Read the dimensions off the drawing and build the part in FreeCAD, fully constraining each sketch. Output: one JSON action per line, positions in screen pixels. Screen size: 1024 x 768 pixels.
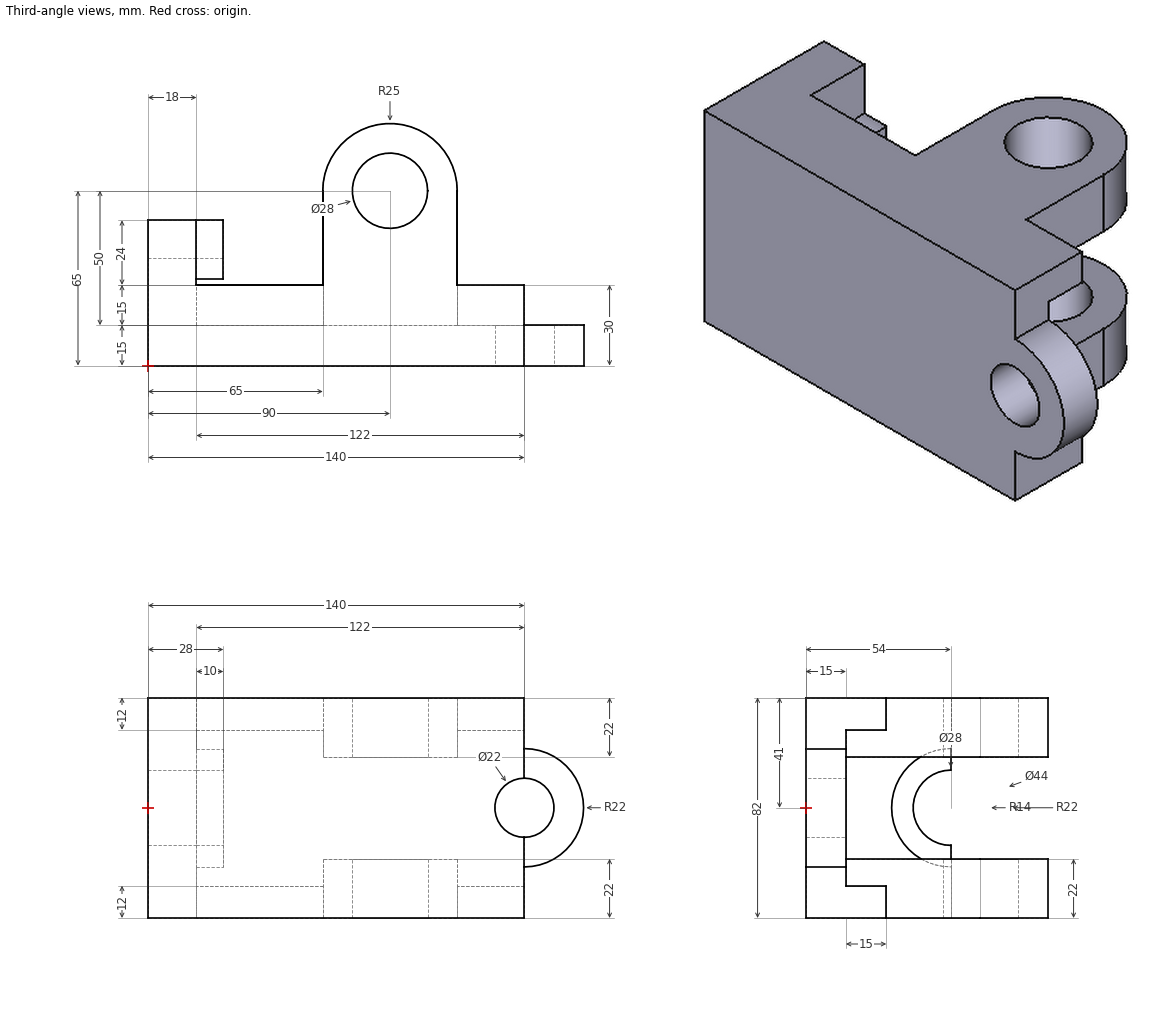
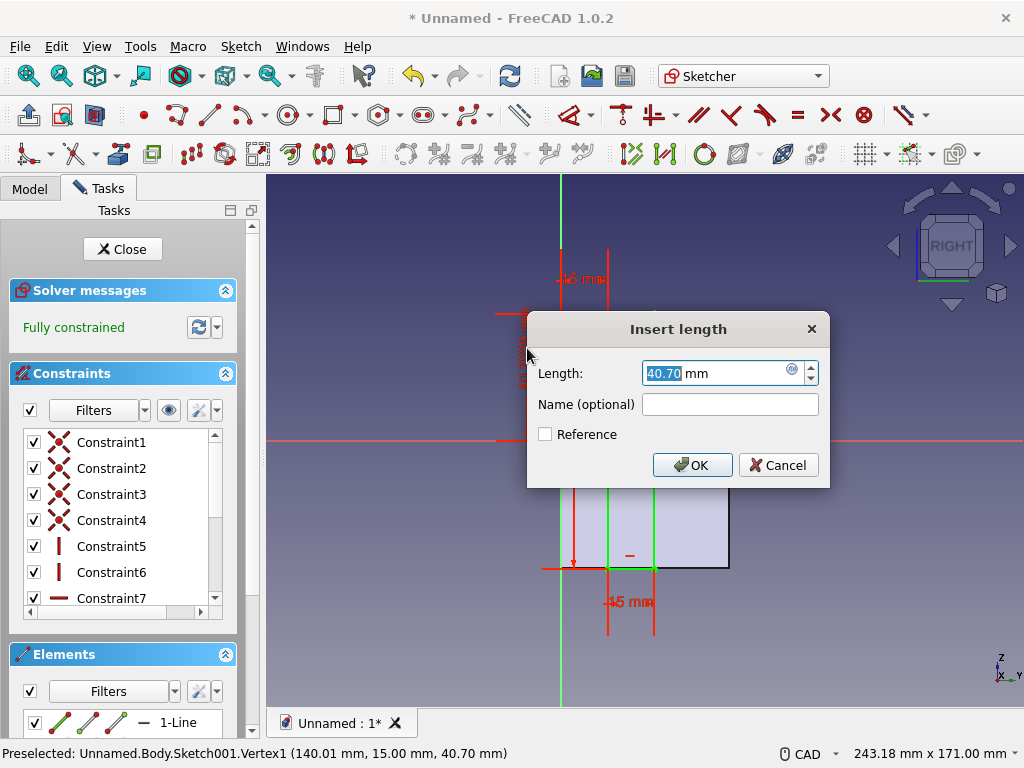
{"action": "type", "text": "41"}
{"action": "key", "text": "Return"}
{"action": "key", "text": "Escape"}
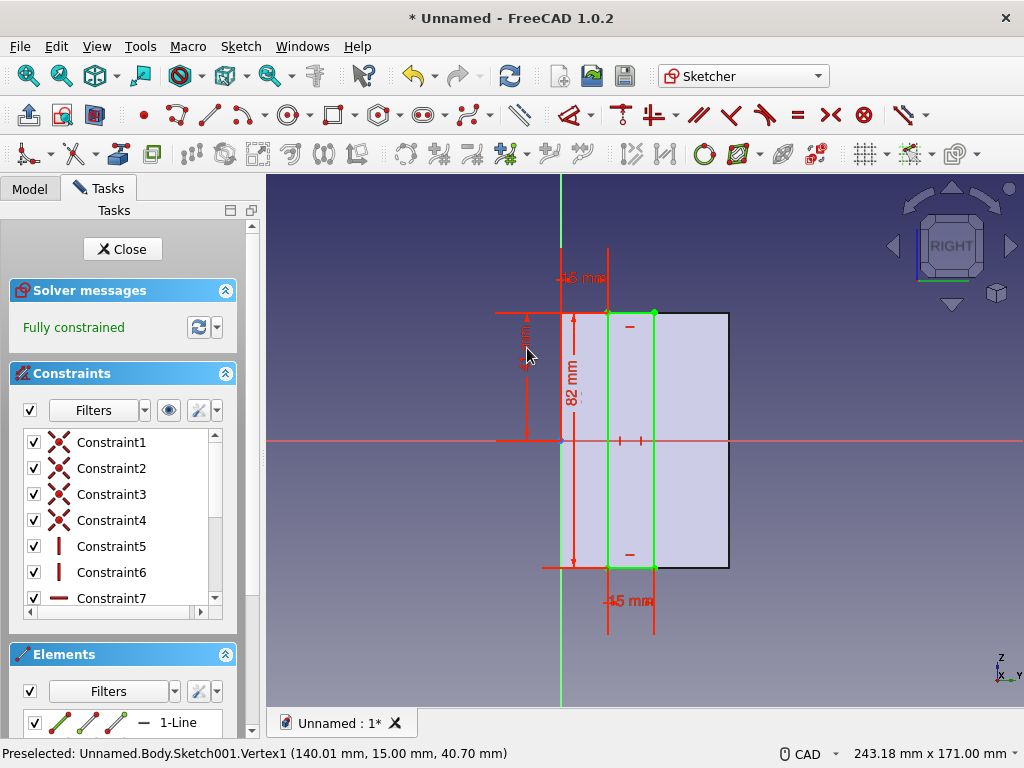
{"action": "left_click", "coordinate": [123, 249]}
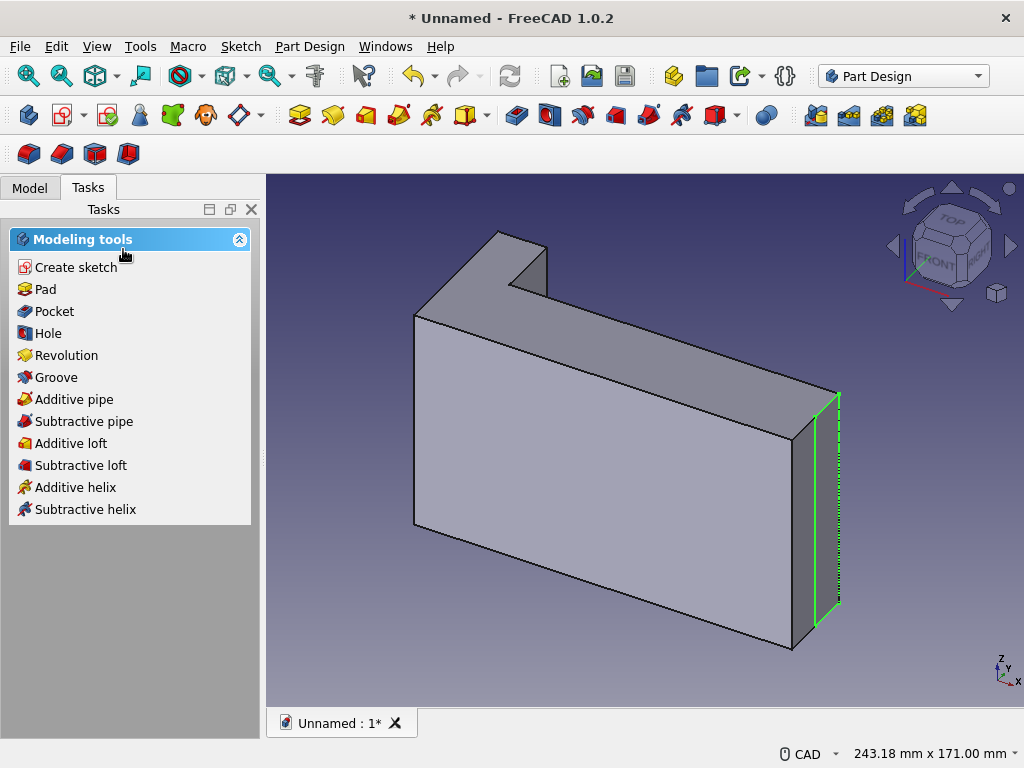
{"action": "left_click", "coordinate": [517, 116]}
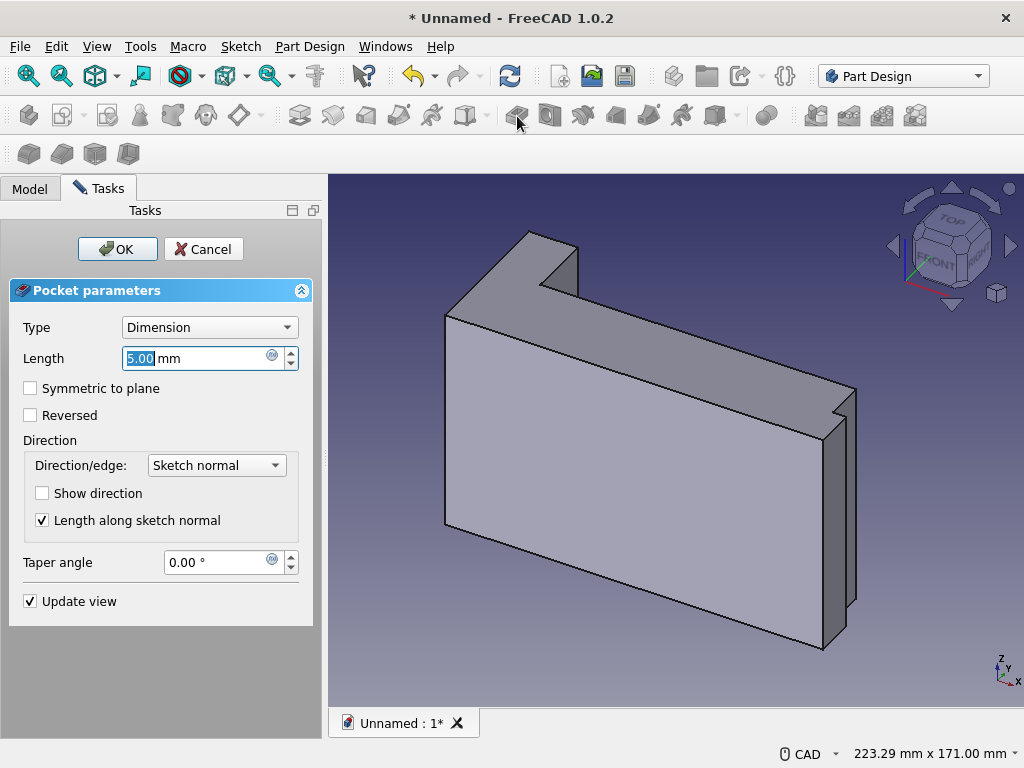
{"action": "type", "text": "122"}
{"action": "key", "text": "Tab"}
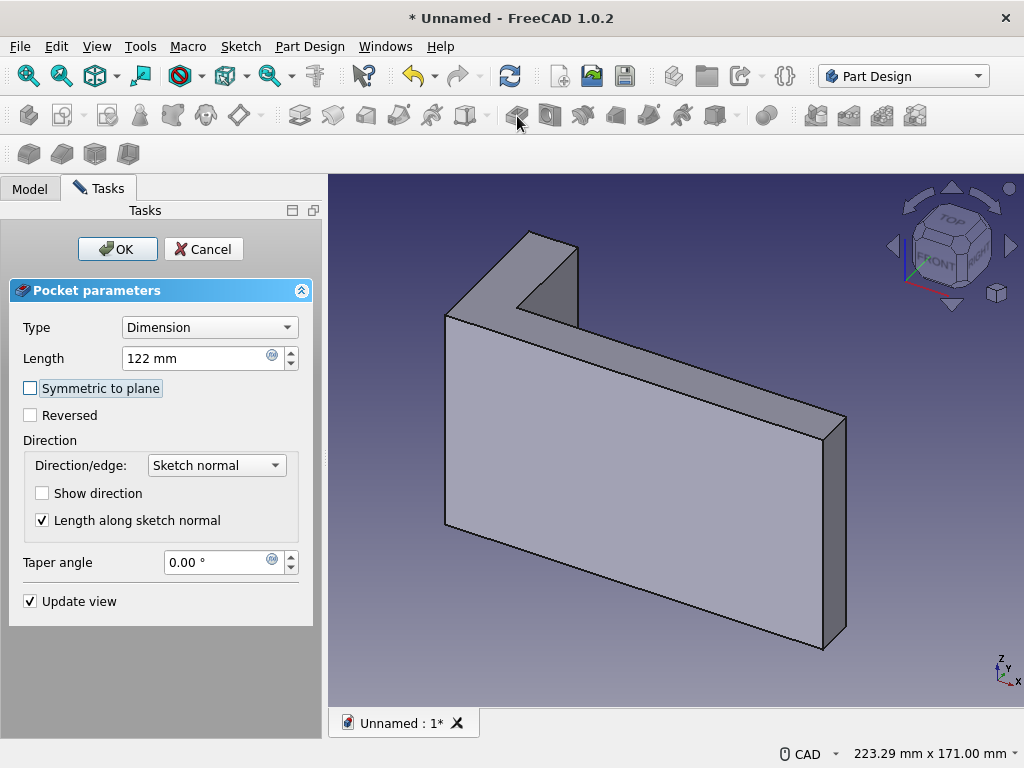
{"action": "left_click", "coordinate": [118, 249]}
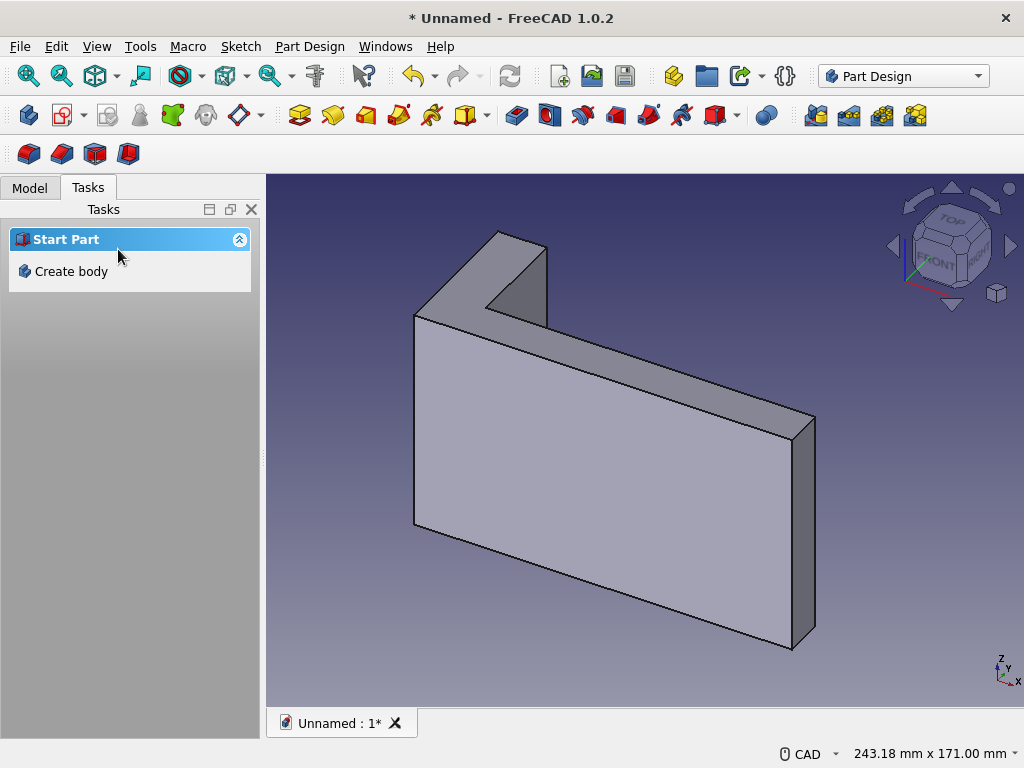
{"action": "left_click", "coordinate": [459, 305]}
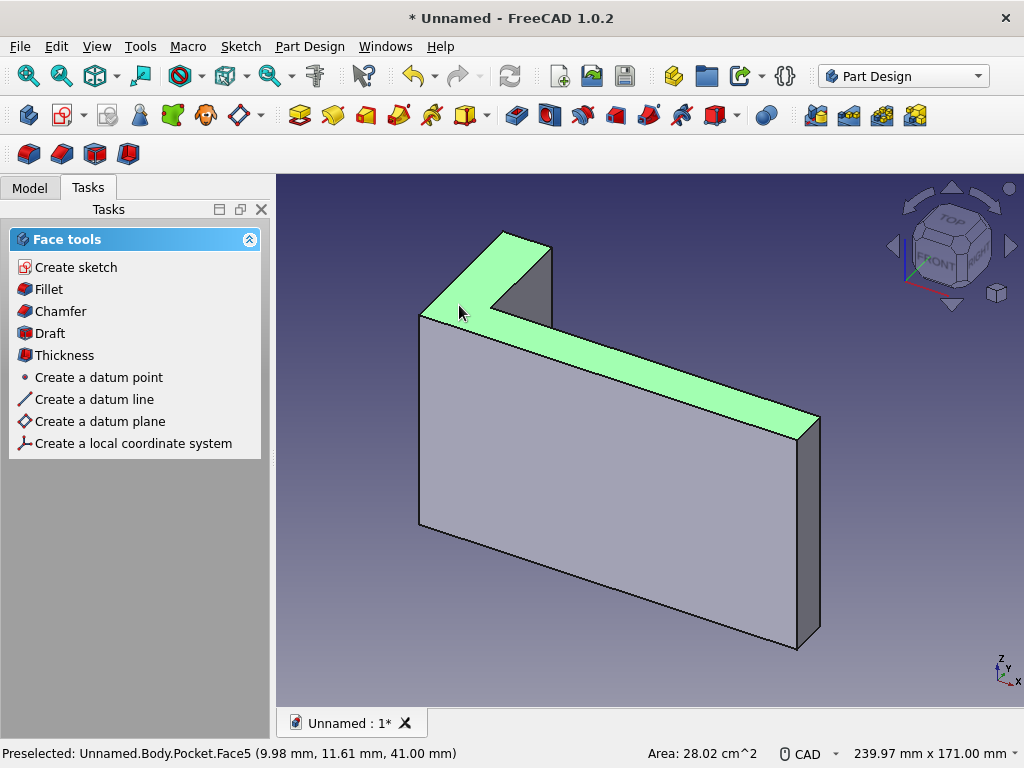
{"action": "left_click", "coordinate": [62, 116]}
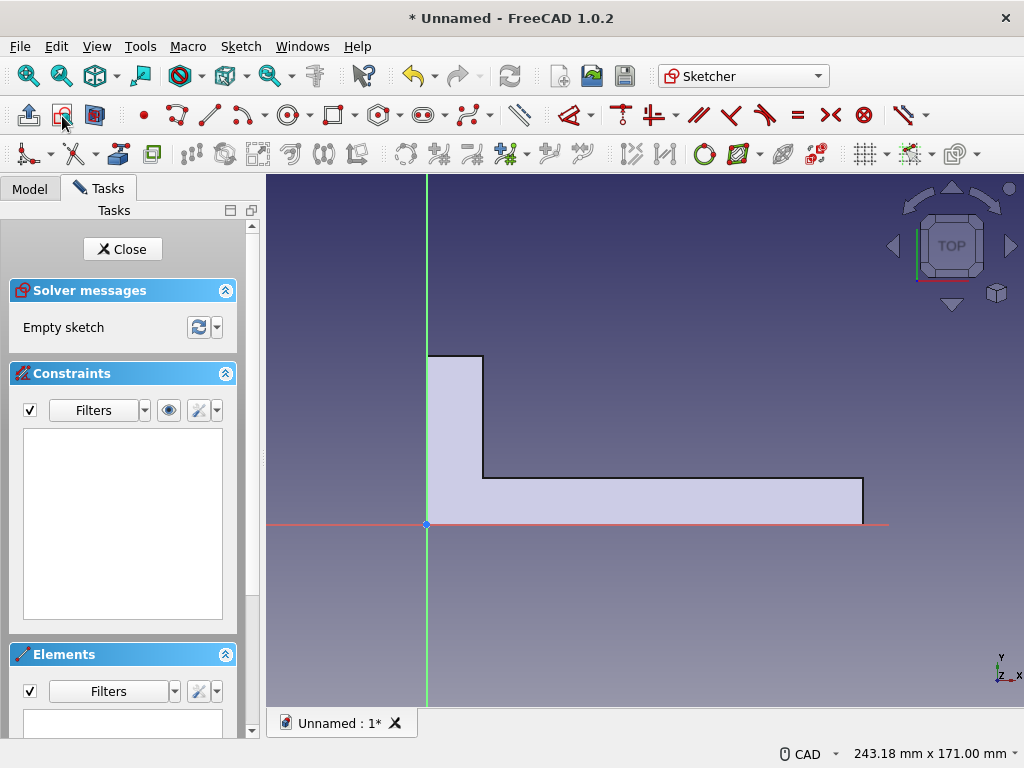
{"action": "scroll", "coordinate": [294, 272], "scroll_direction": "down", "scroll_amount": 1}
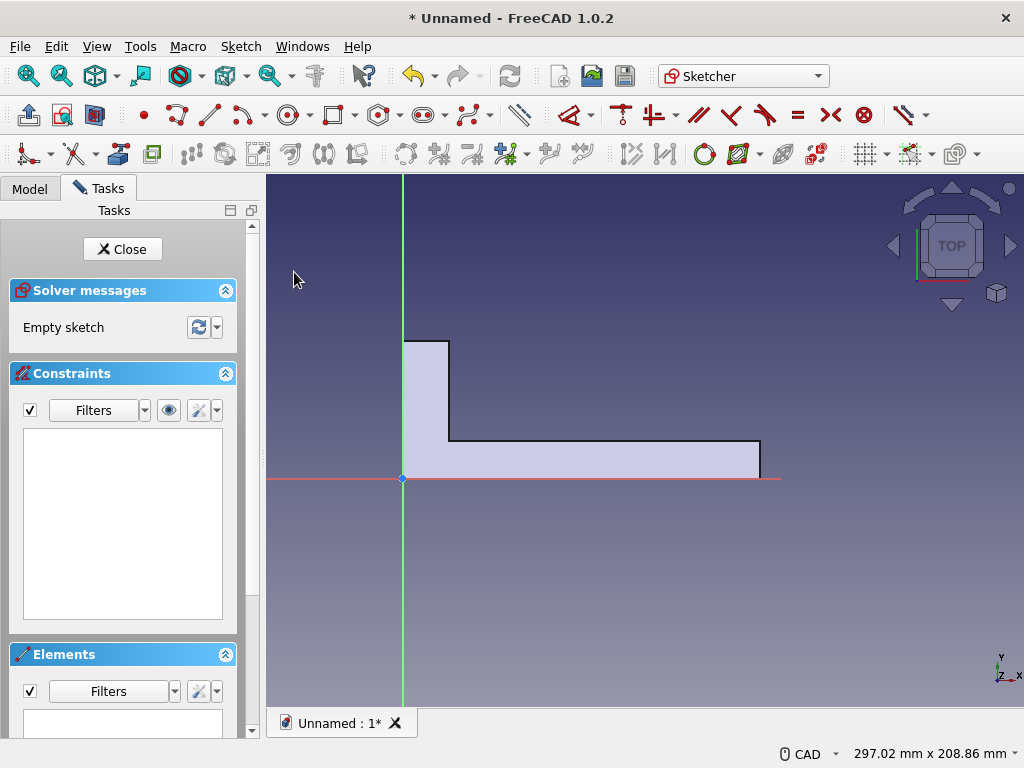
{"action": "key", "text": "g r"}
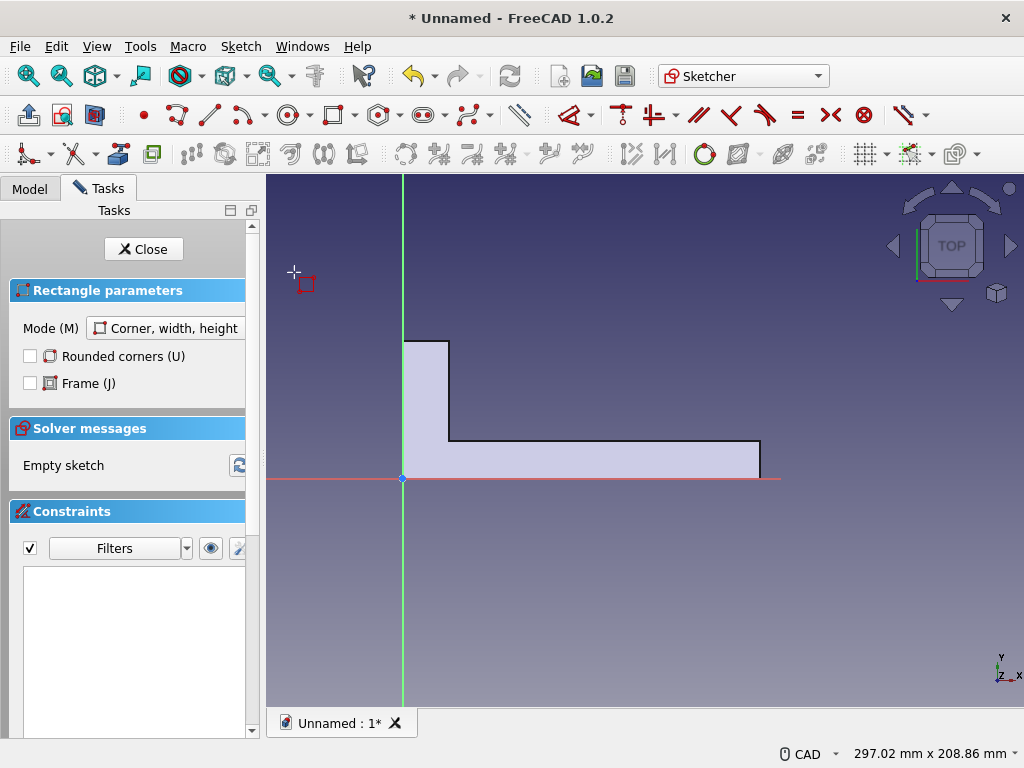
{"action": "left_click", "coordinate": [449, 402]}
{"action": "left_click", "coordinate": [760, 441]}
{"action": "key", "text": "Escape"}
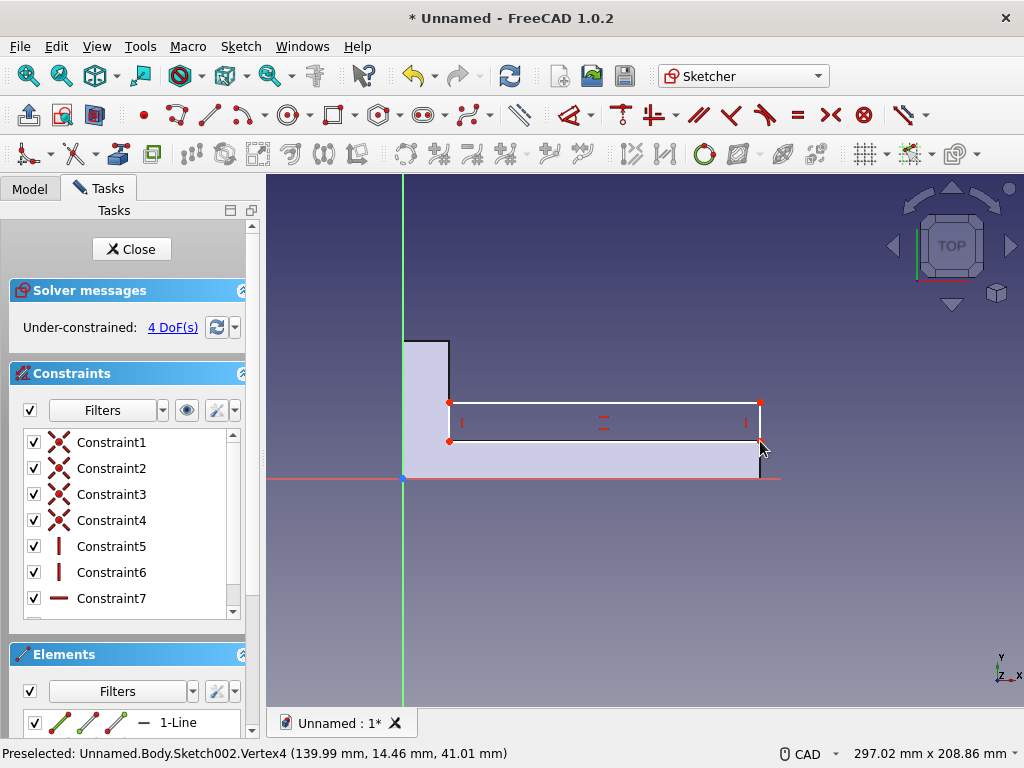
{"action": "left_click", "coordinate": [568, 116]}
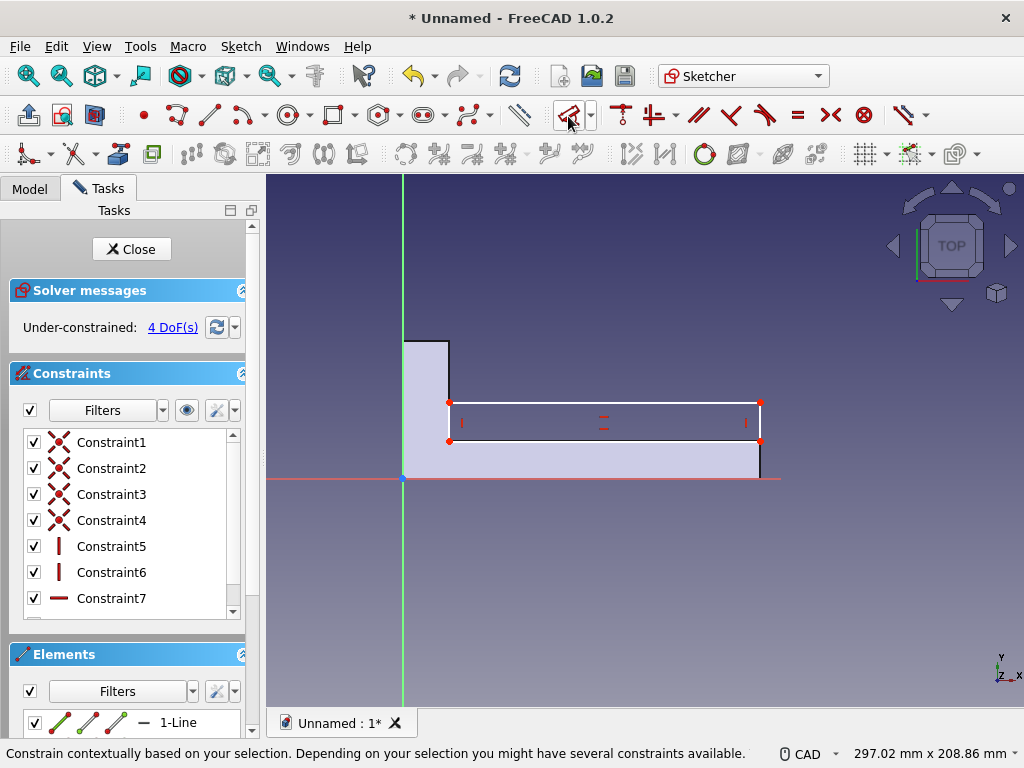
{"action": "left_click", "coordinate": [449, 415]}
{"action": "left_click", "coordinate": [483, 422]}